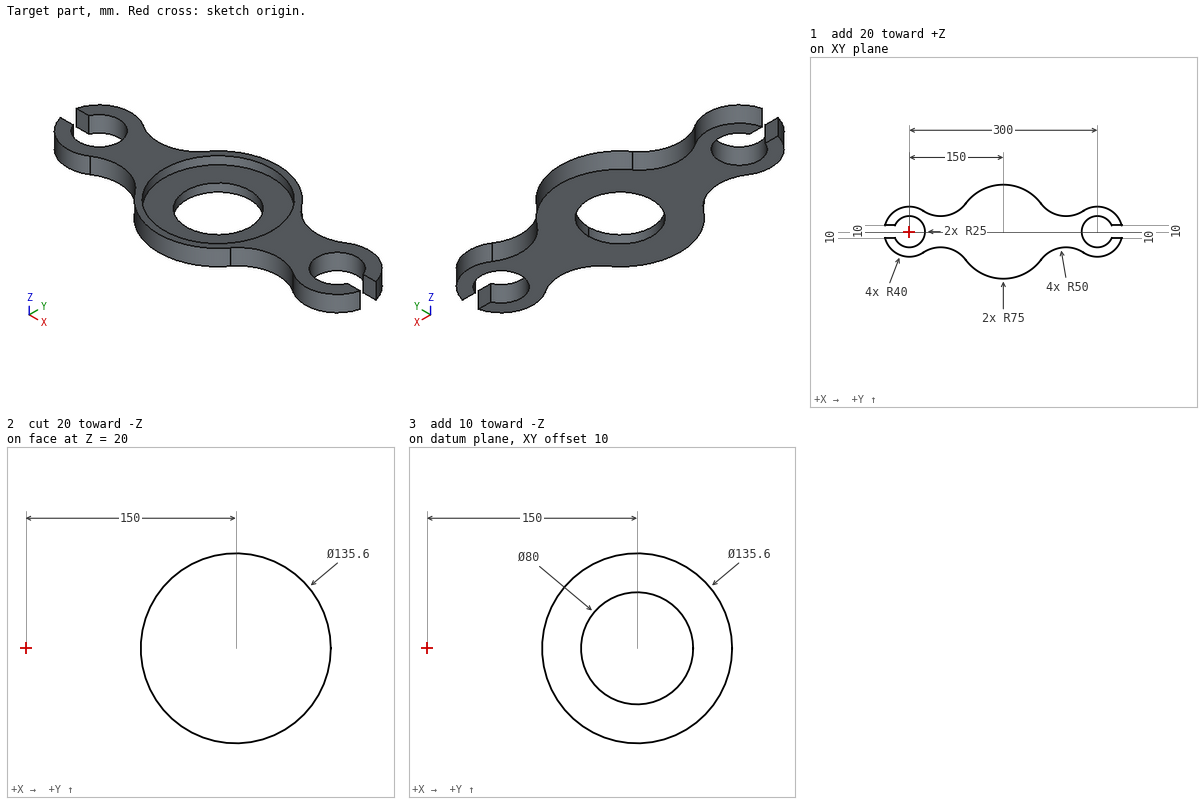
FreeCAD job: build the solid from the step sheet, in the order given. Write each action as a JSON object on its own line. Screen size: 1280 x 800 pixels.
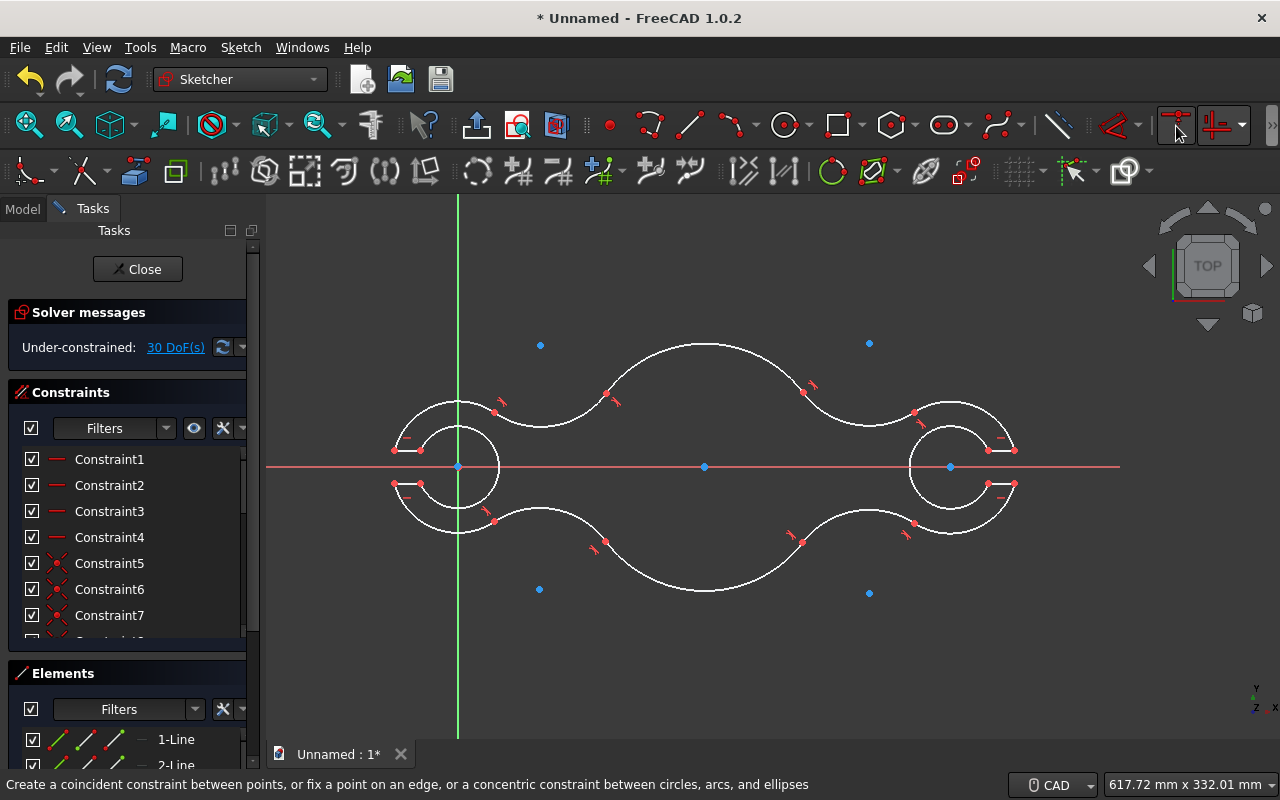
{"action": "left_click", "coordinate": [950, 534]}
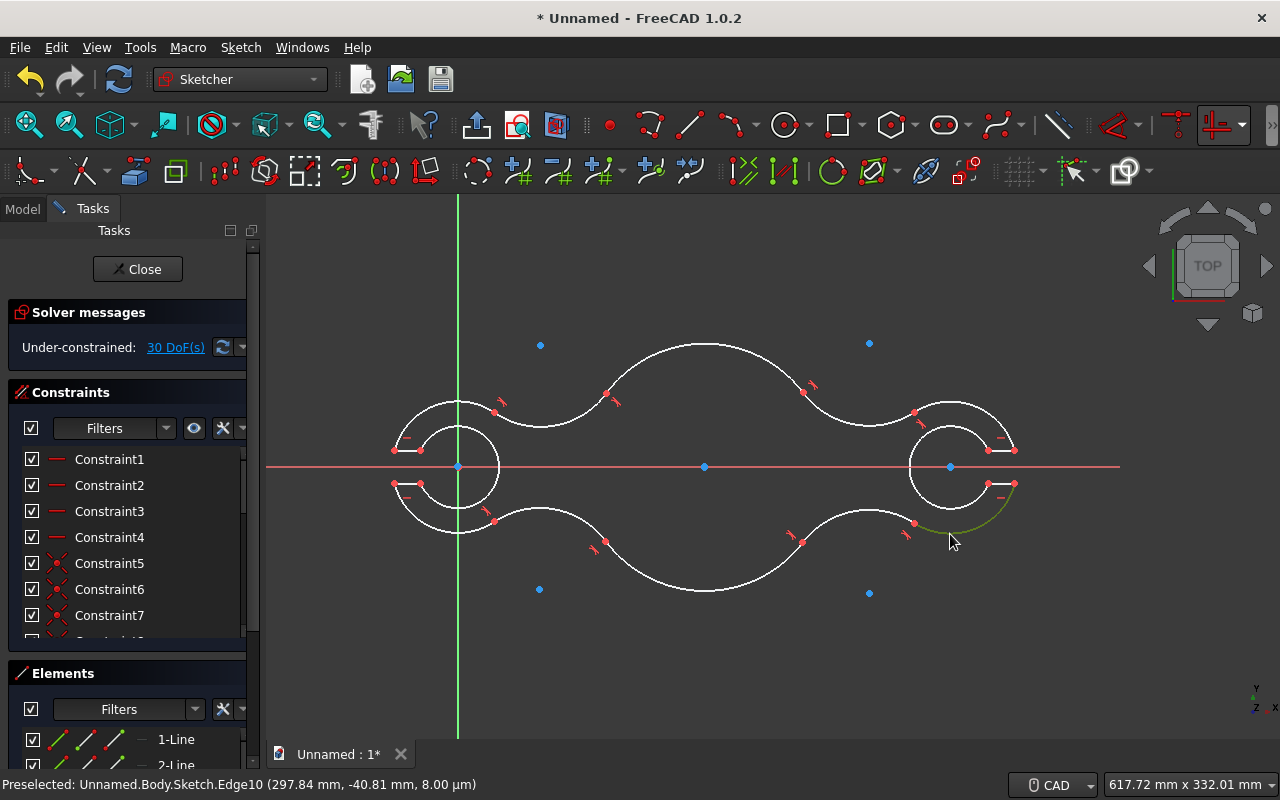
{"action": "left_click", "coordinate": [932, 431]}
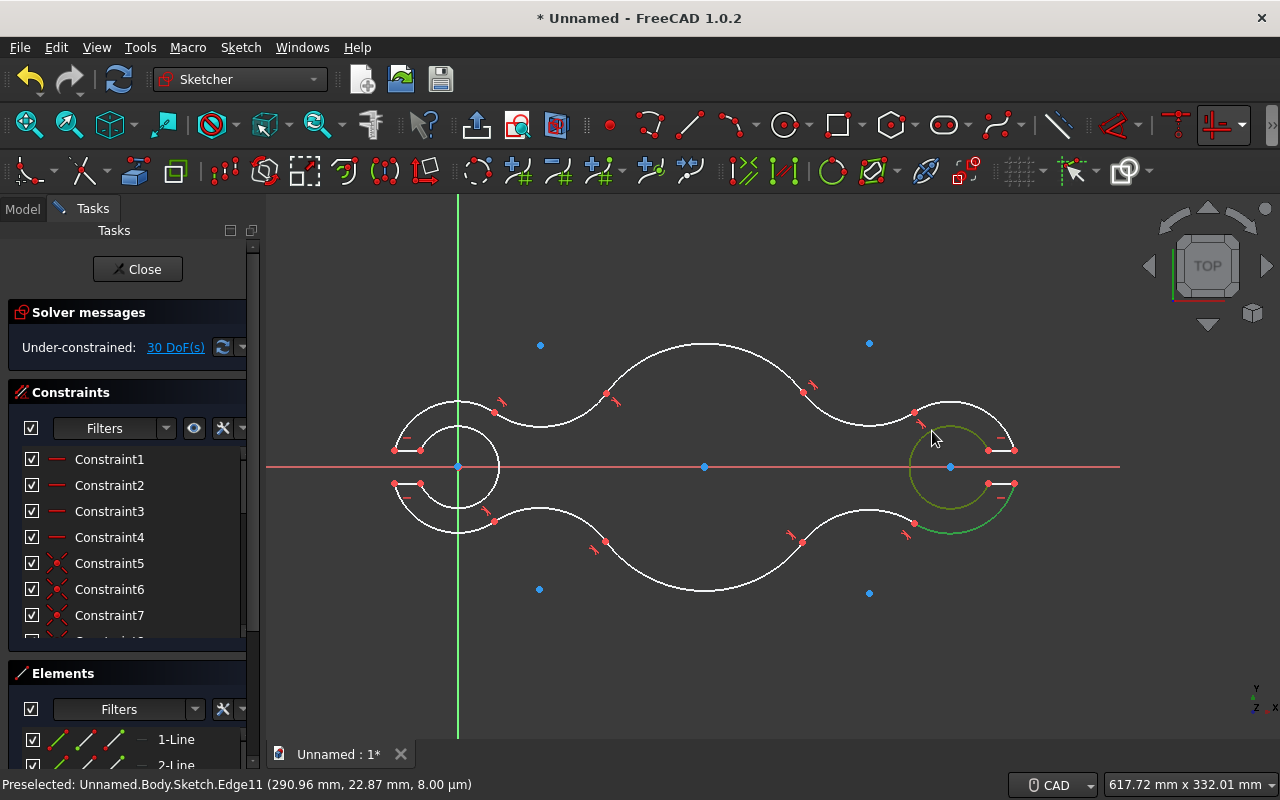
{"action": "left_click", "coordinate": [1176, 126]}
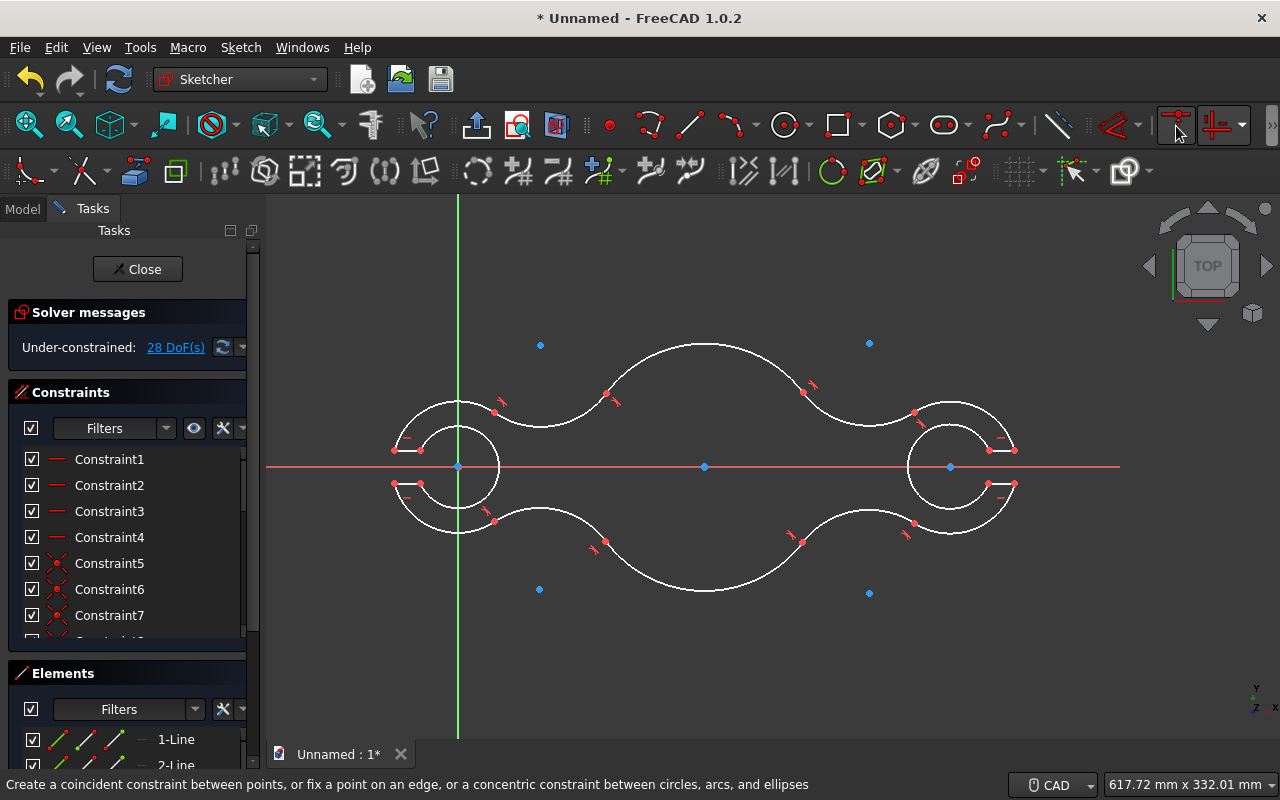
{"action": "left_click", "coordinate": [950, 534]}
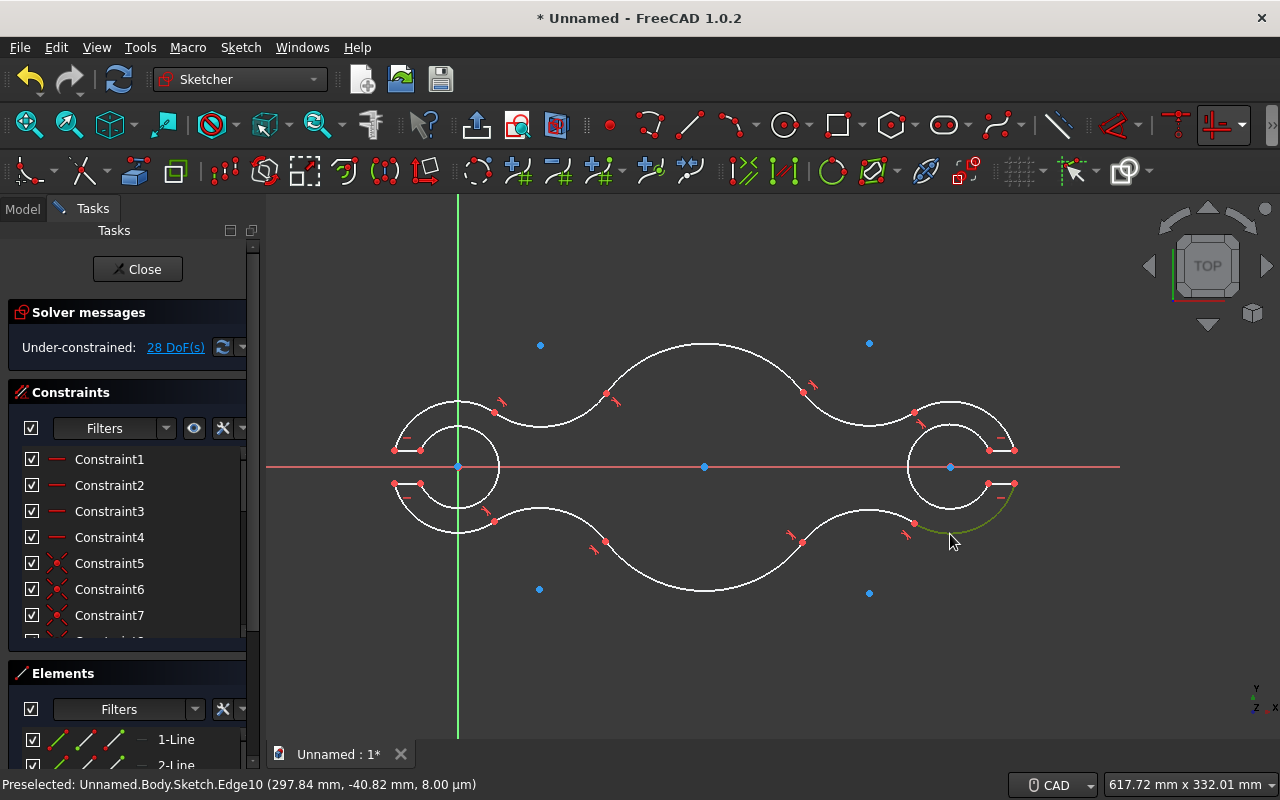
{"action": "left_click", "coordinate": [996, 419]}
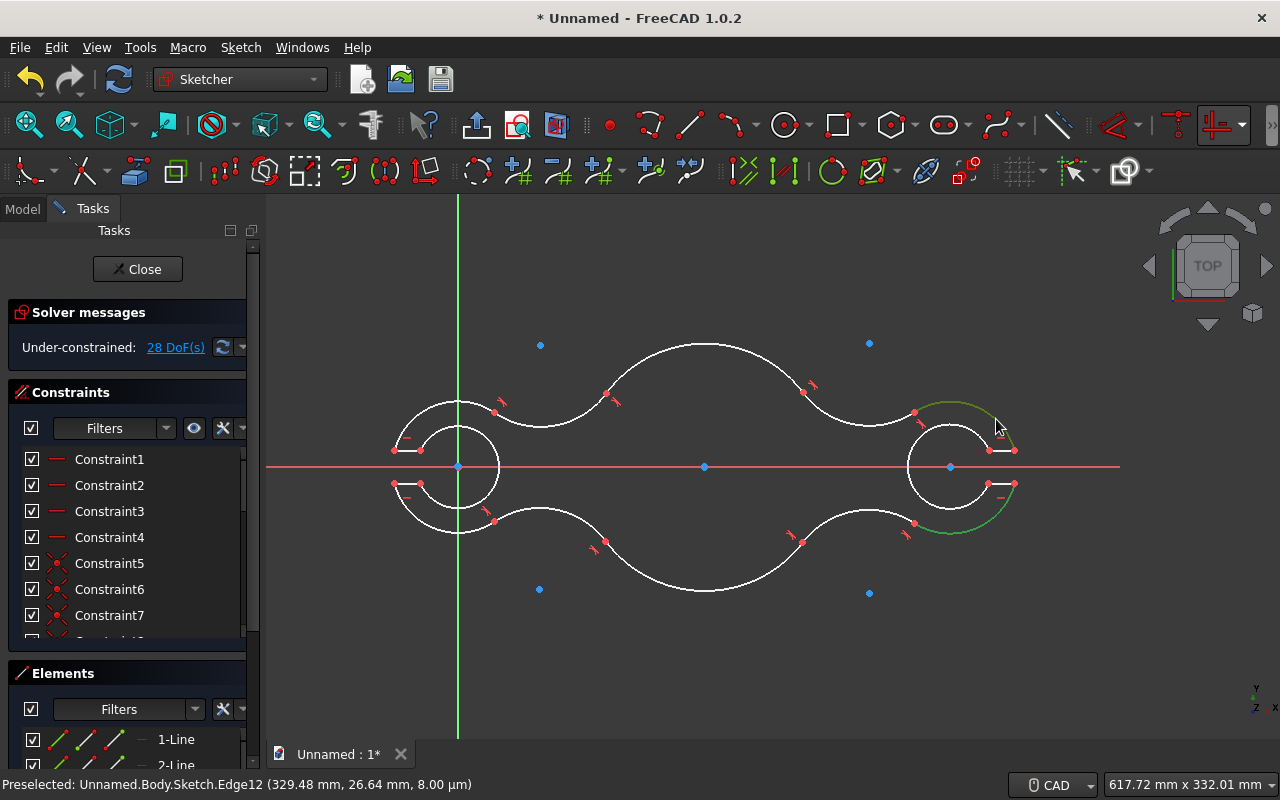
{"action": "left_click", "coordinate": [1176, 126]}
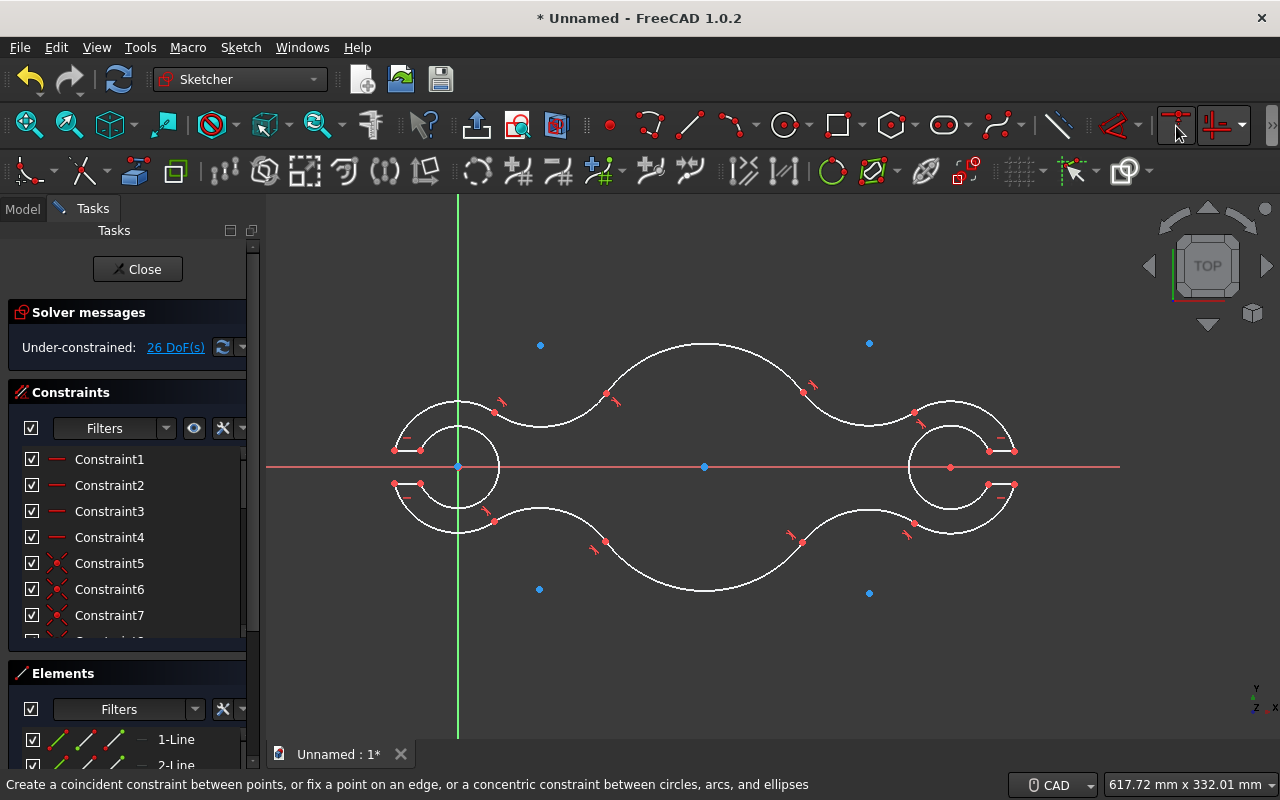
{"action": "left_click", "coordinate": [659, 582]}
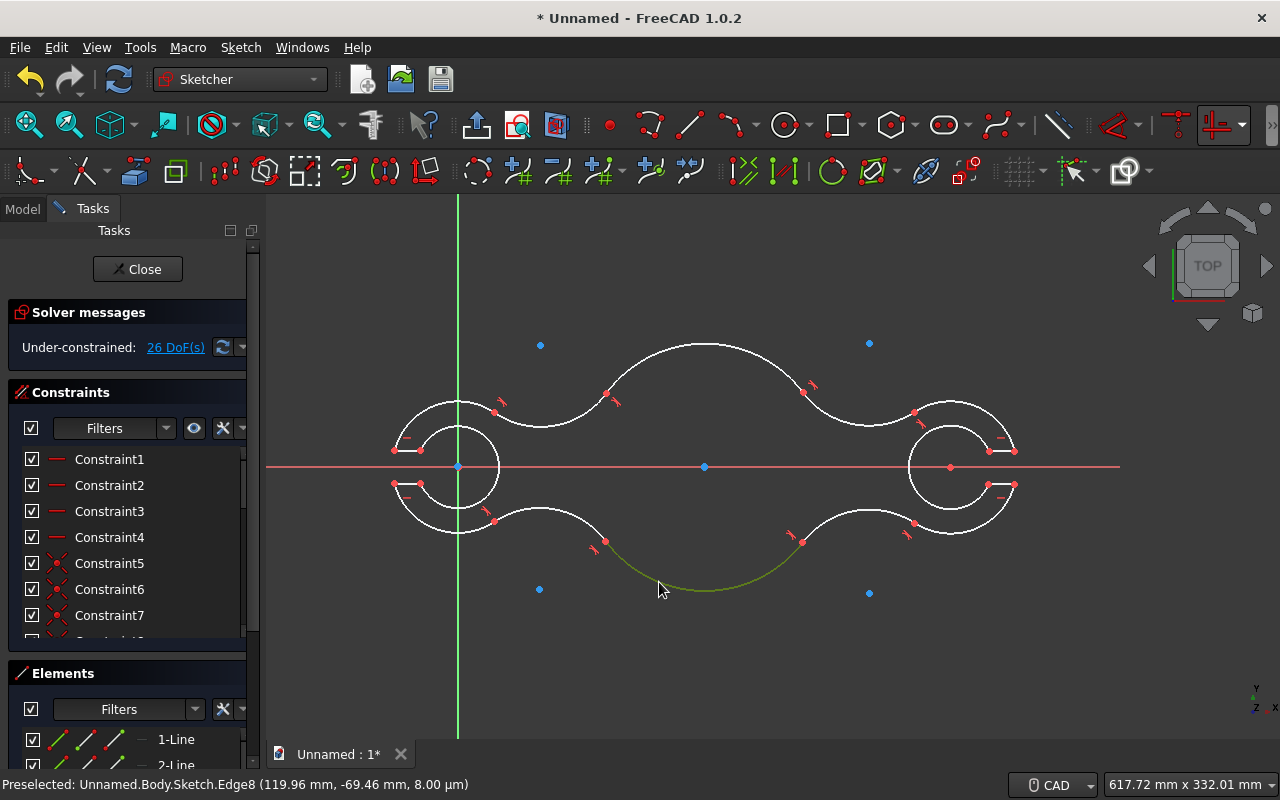
{"action": "left_click", "coordinate": [749, 352]}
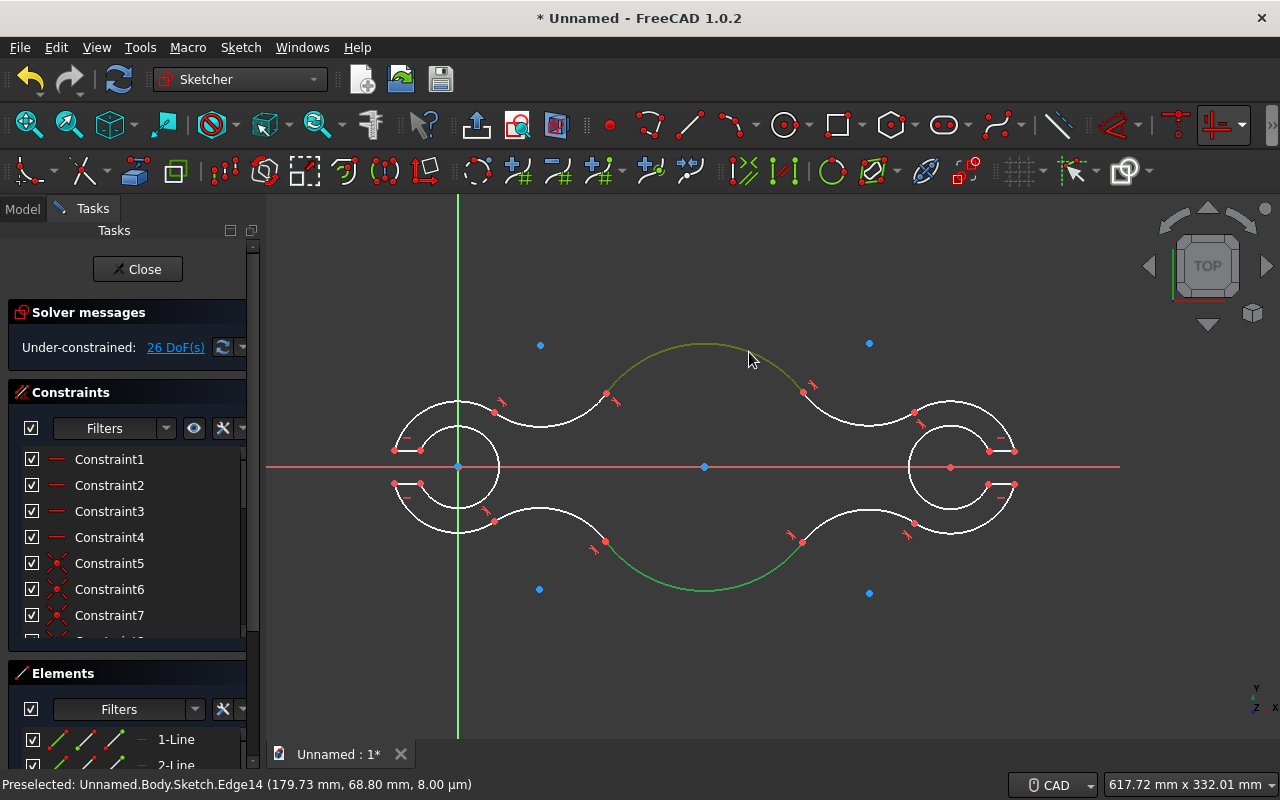
{"action": "left_click", "coordinate": [1176, 126]}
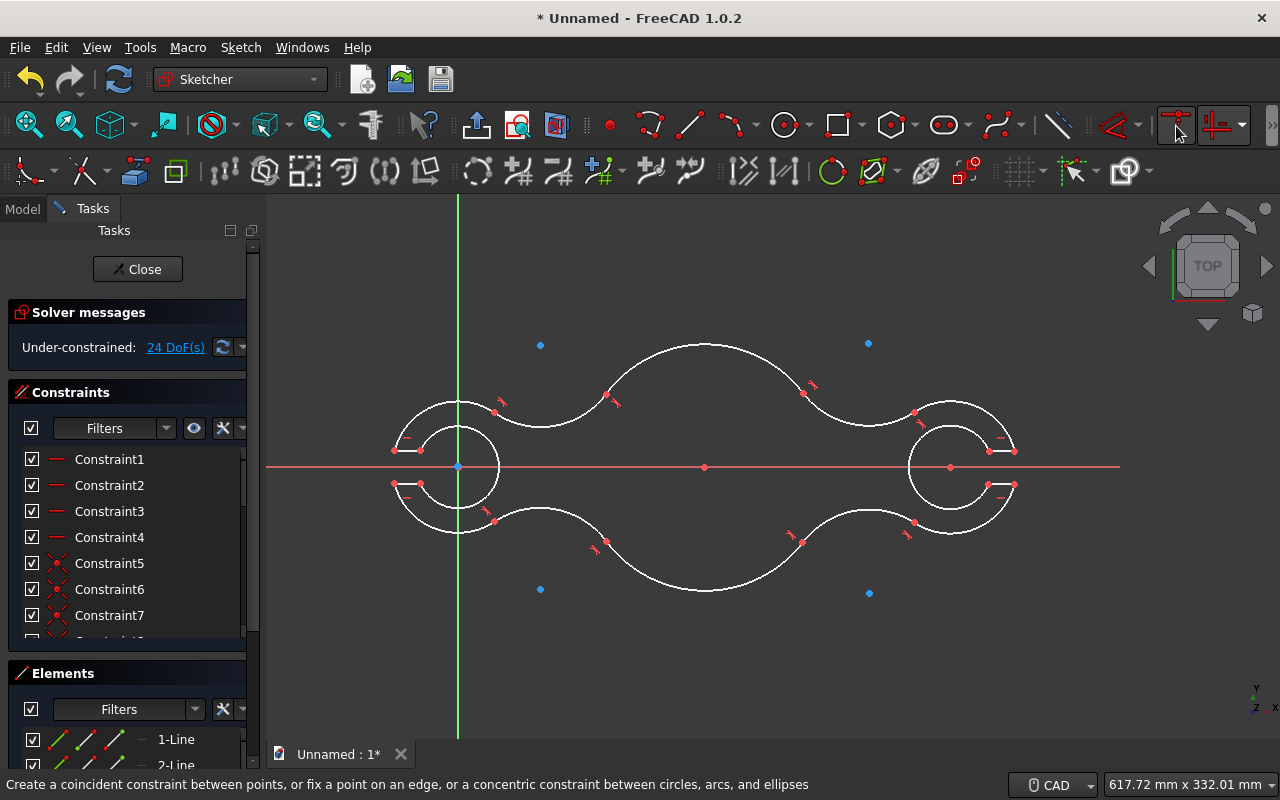
{"action": "left_click", "coordinate": [477, 503]}